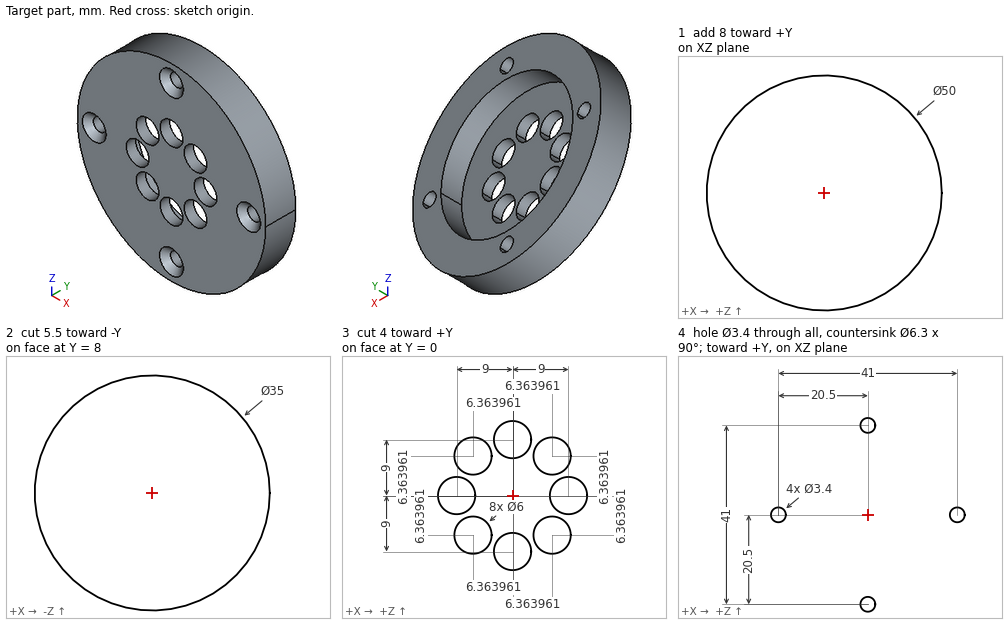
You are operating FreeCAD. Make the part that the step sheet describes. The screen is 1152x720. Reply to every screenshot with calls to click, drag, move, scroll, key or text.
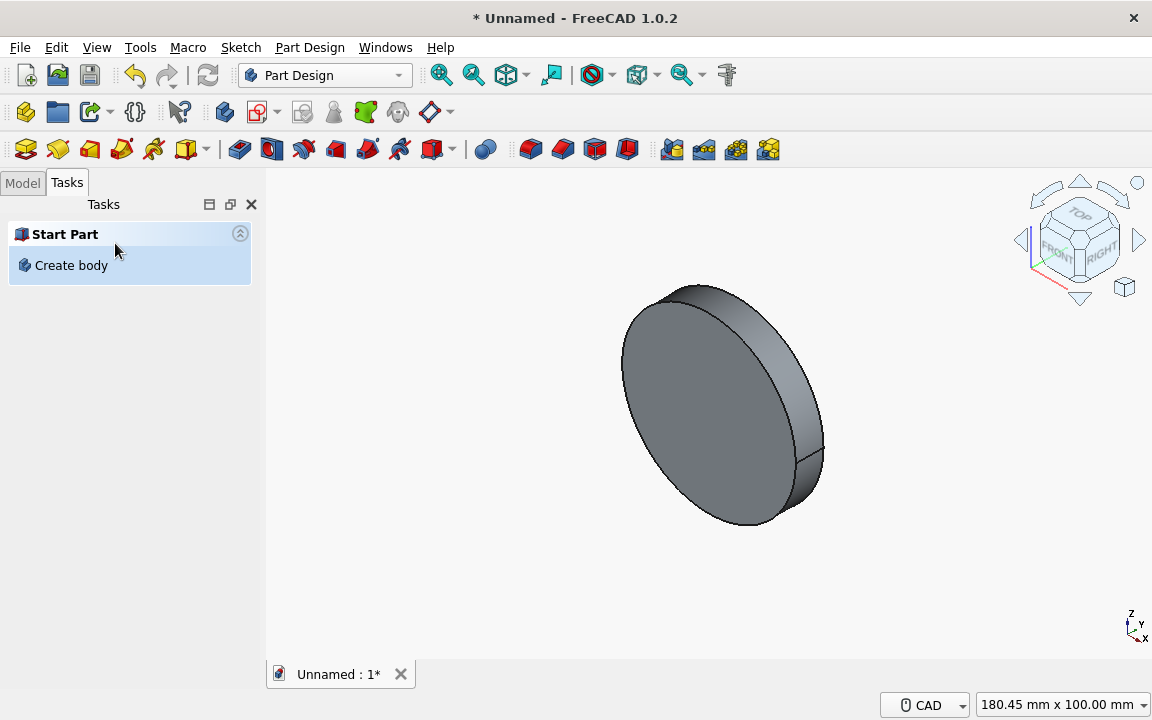
click(709, 412)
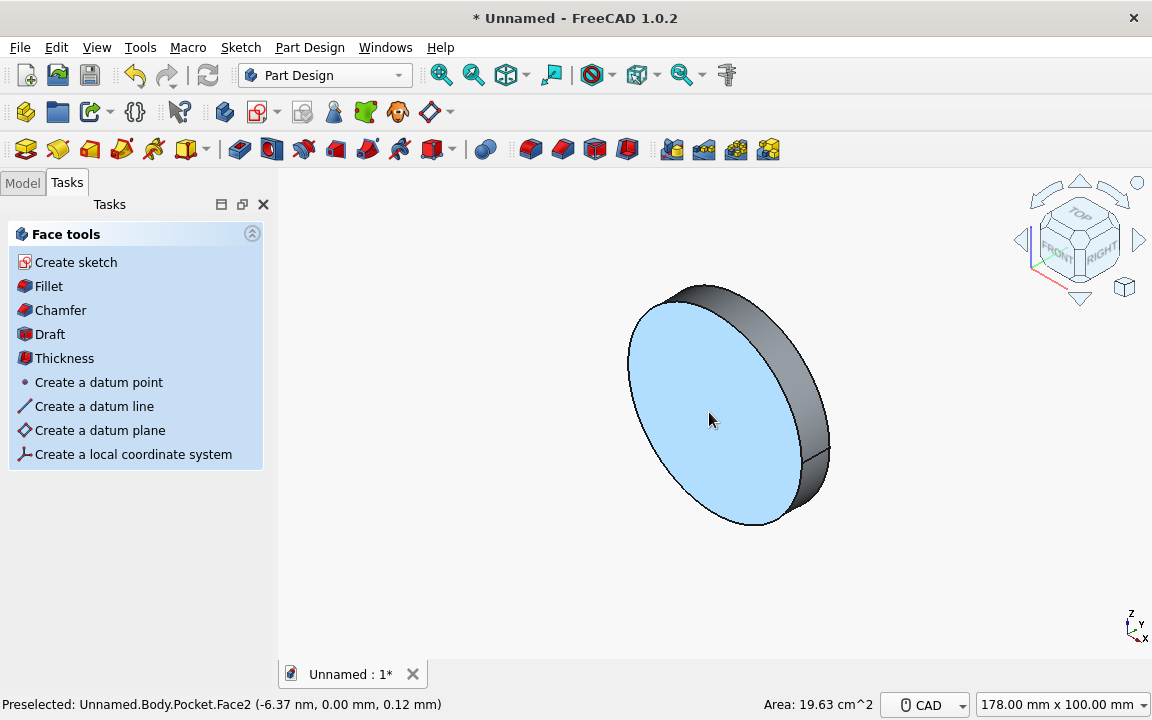
click(258, 112)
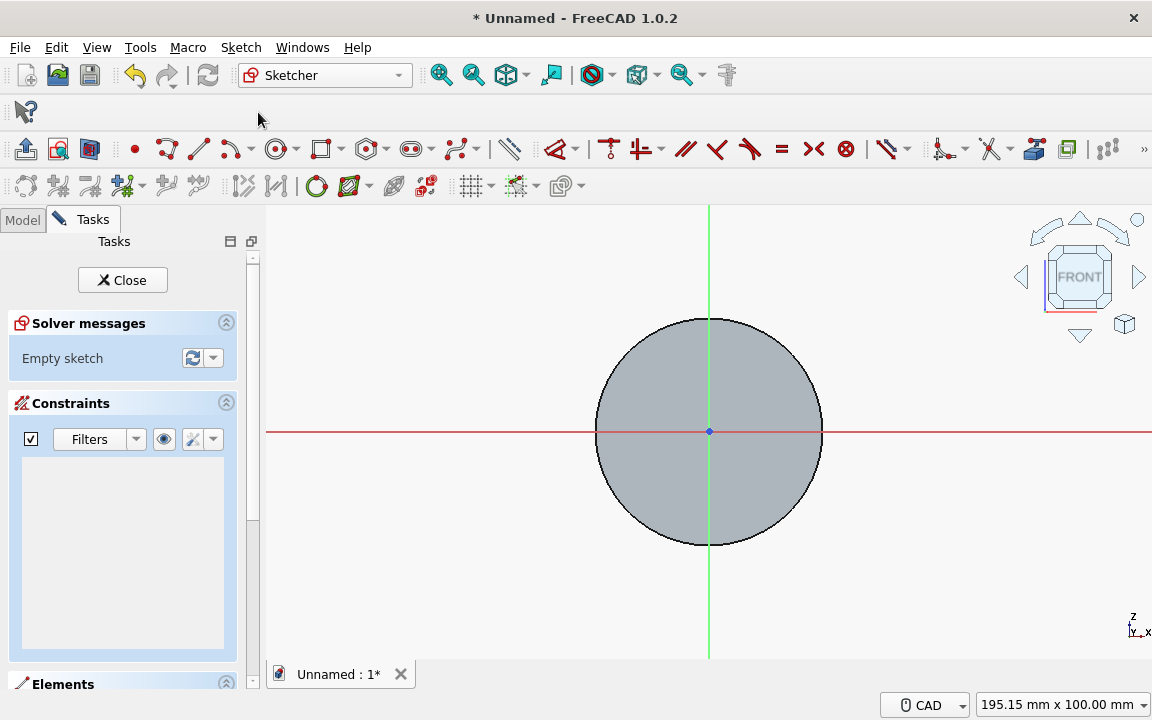
scroll(749, 432, up, 5)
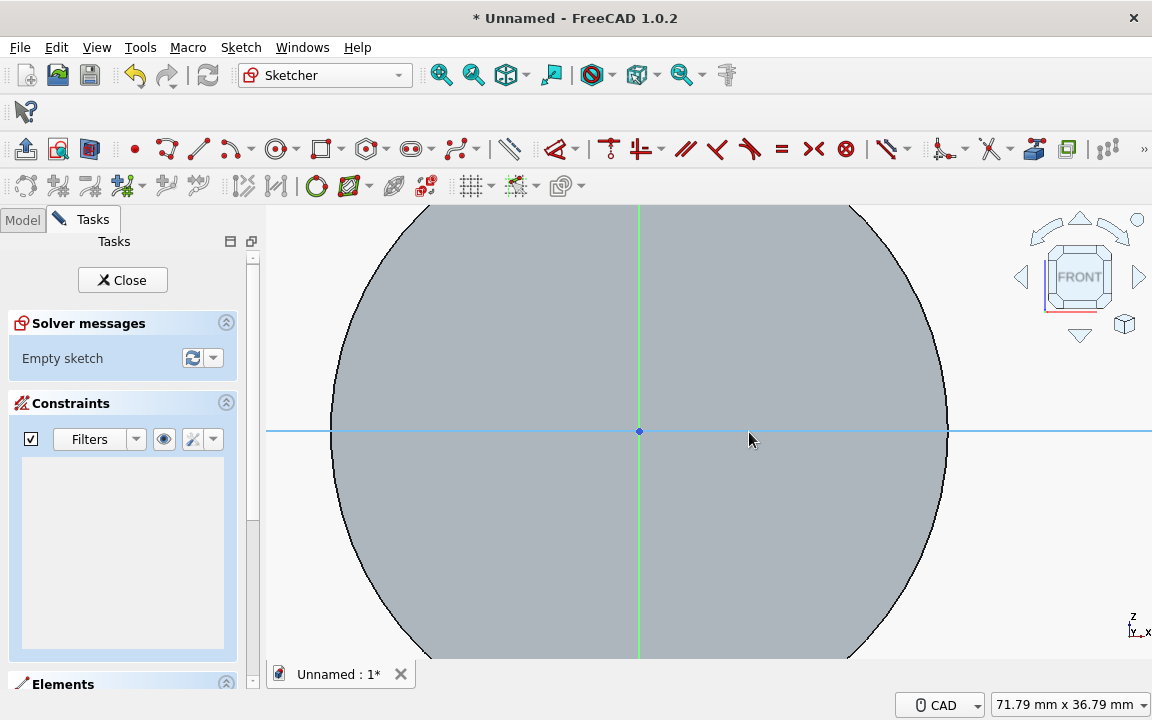
click(276, 150)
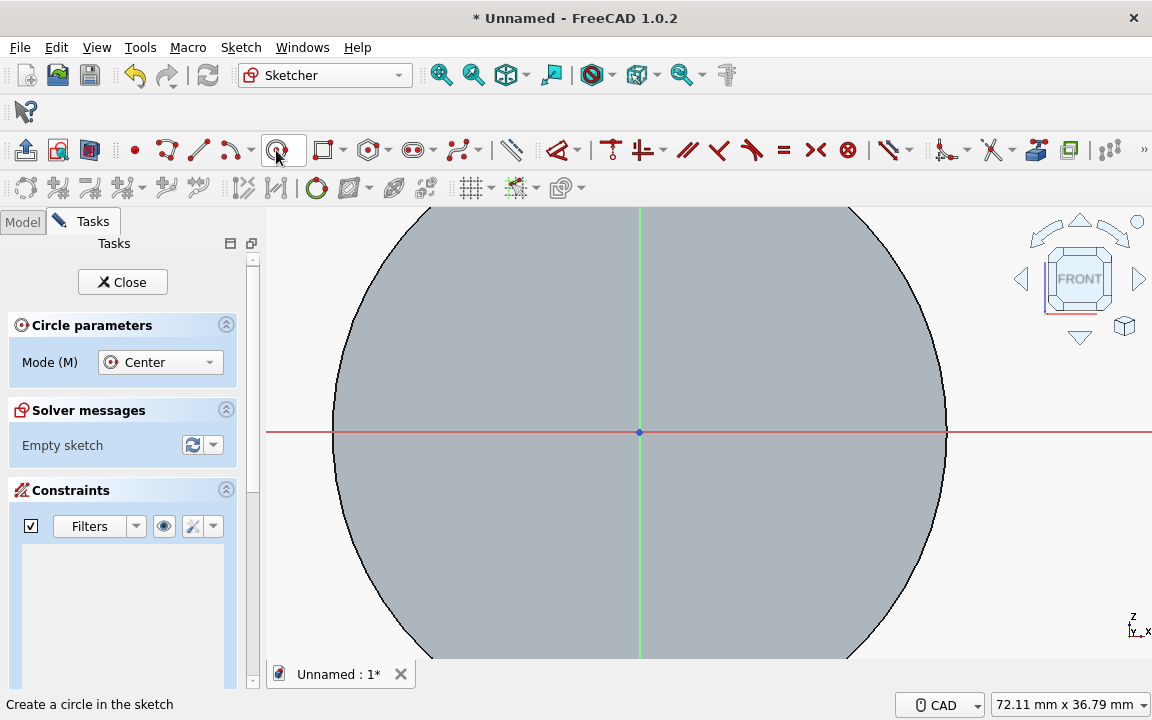
click(640, 543)
move(666, 517)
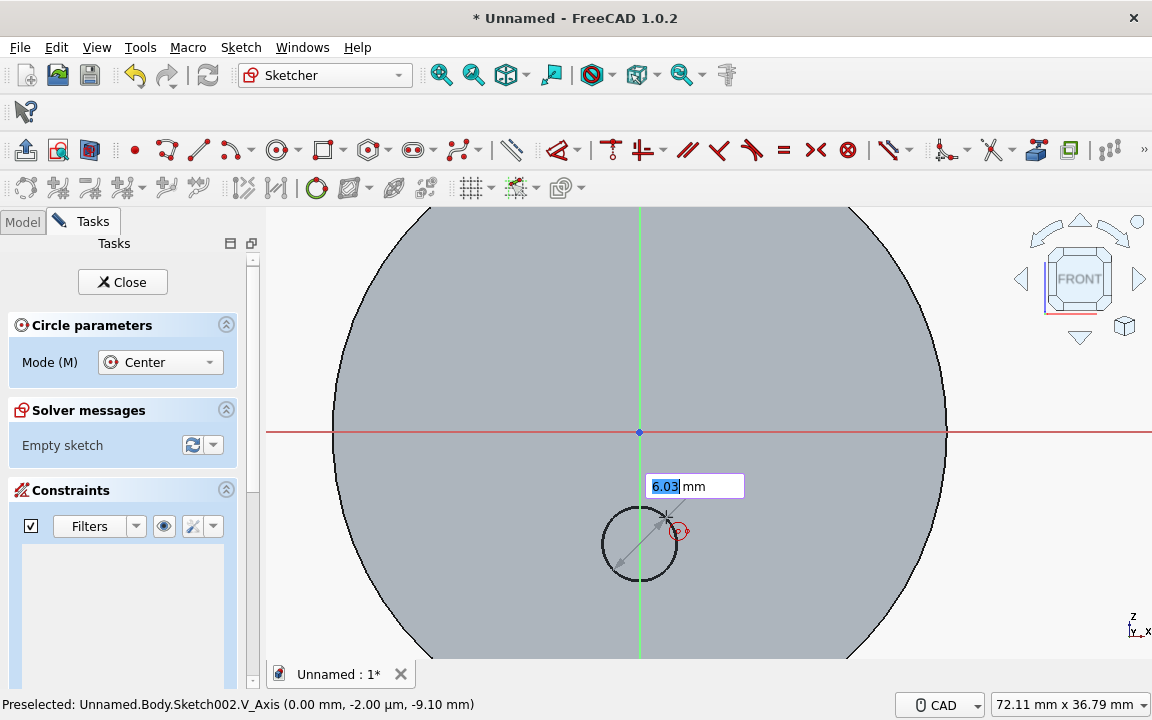
text(6)
key(Return)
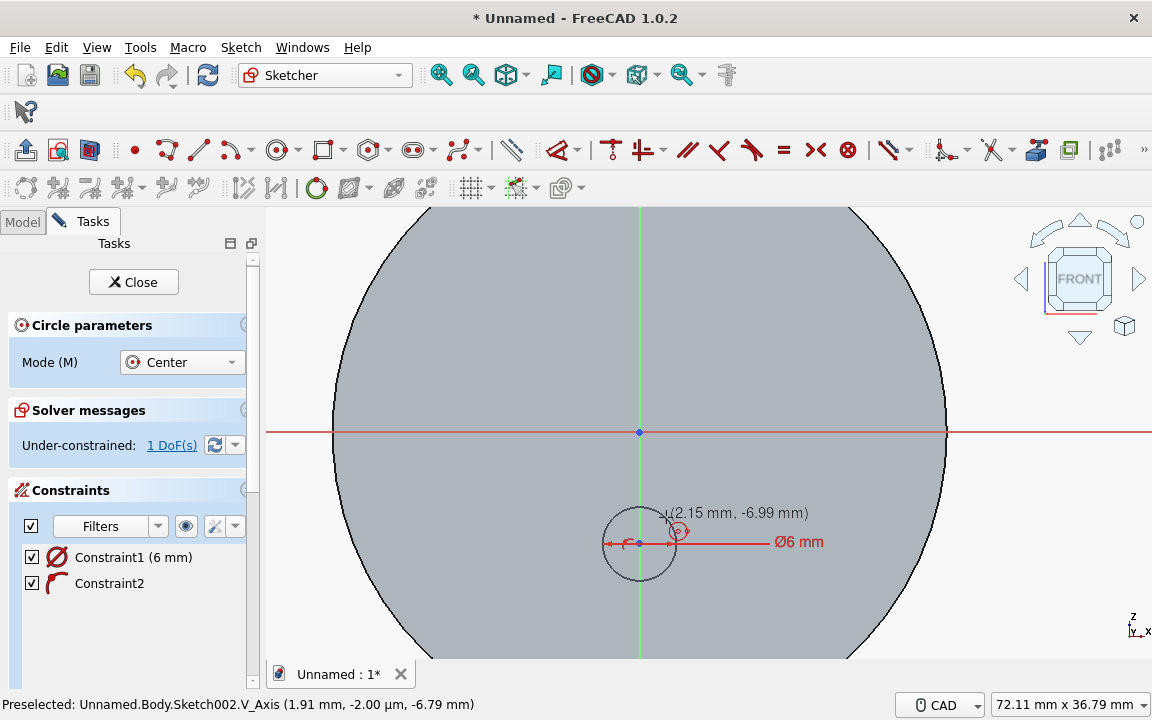
click(561, 510)
move(588, 484)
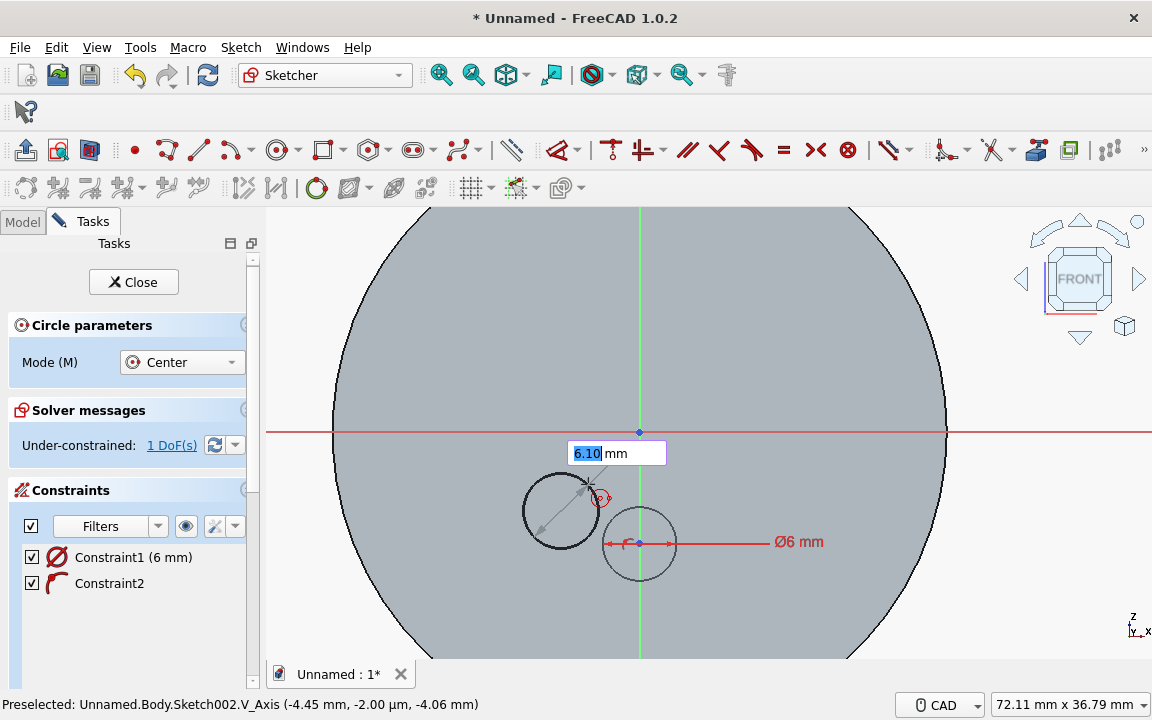
text(6)
key(Return)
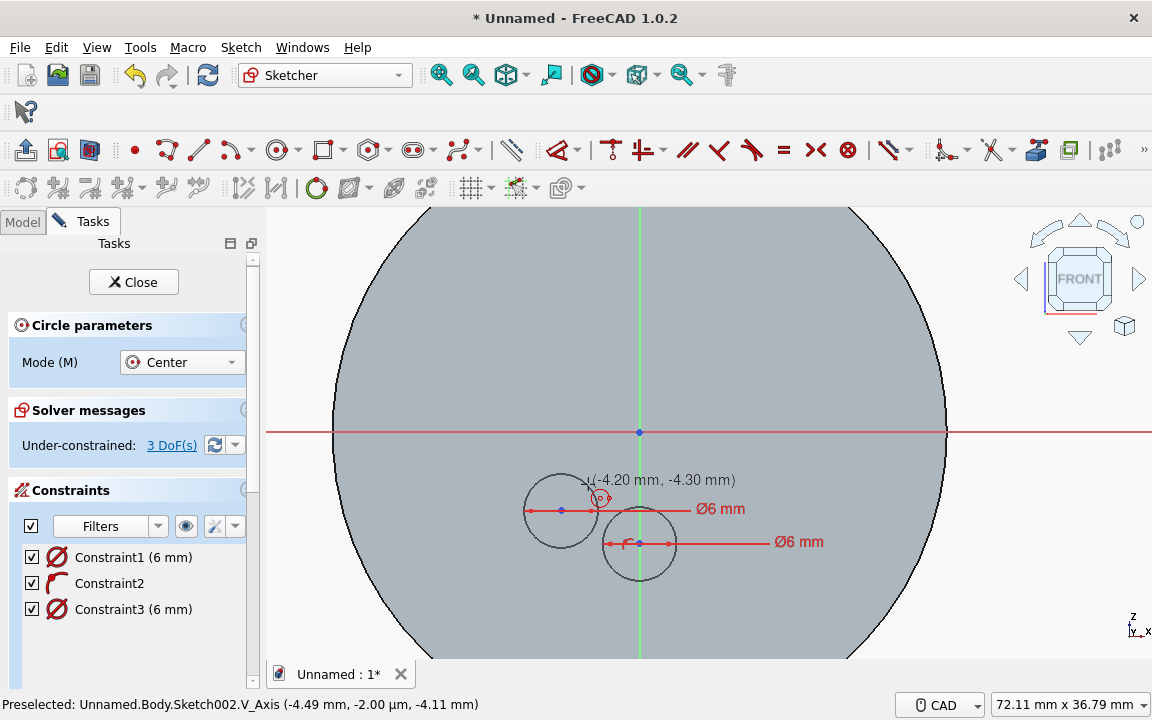
click(529, 432)
move(555, 406)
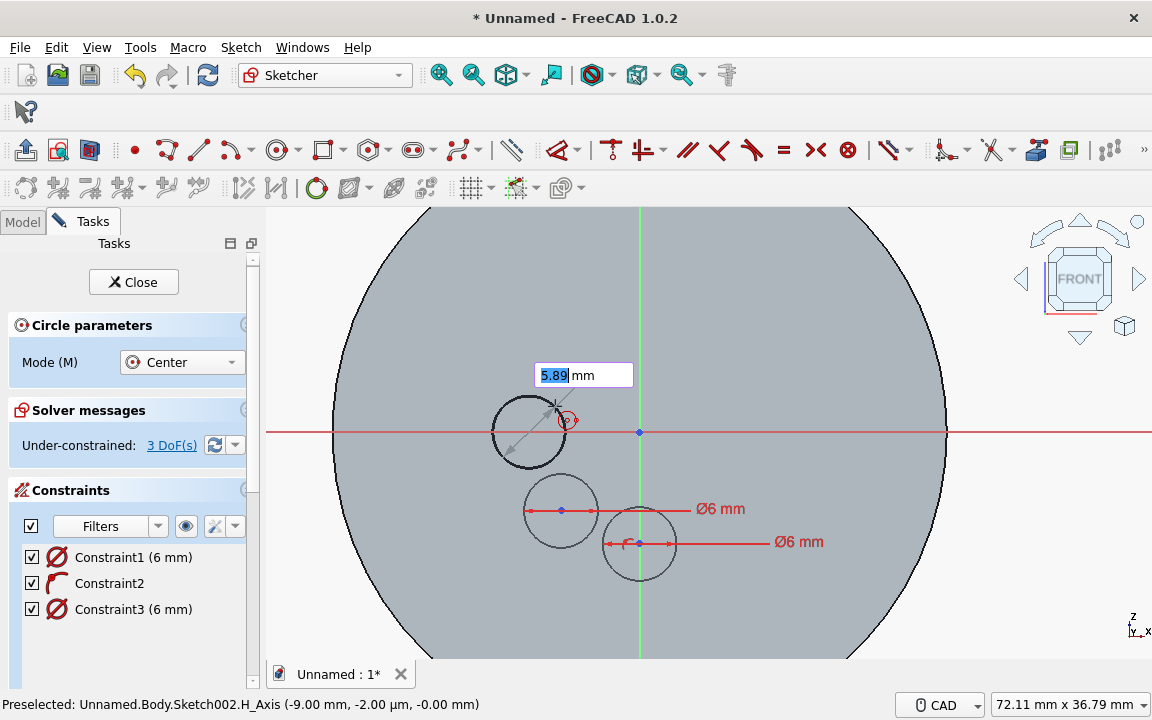
text(6)
key(Return)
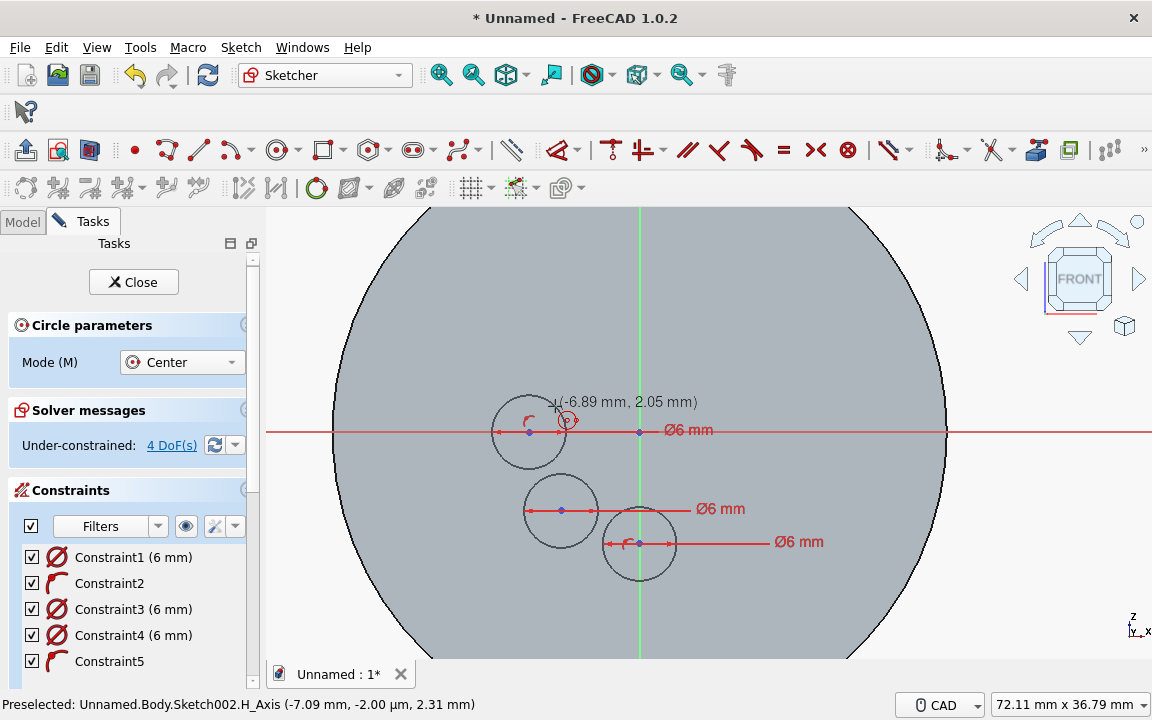
click(561, 354)
move(588, 328)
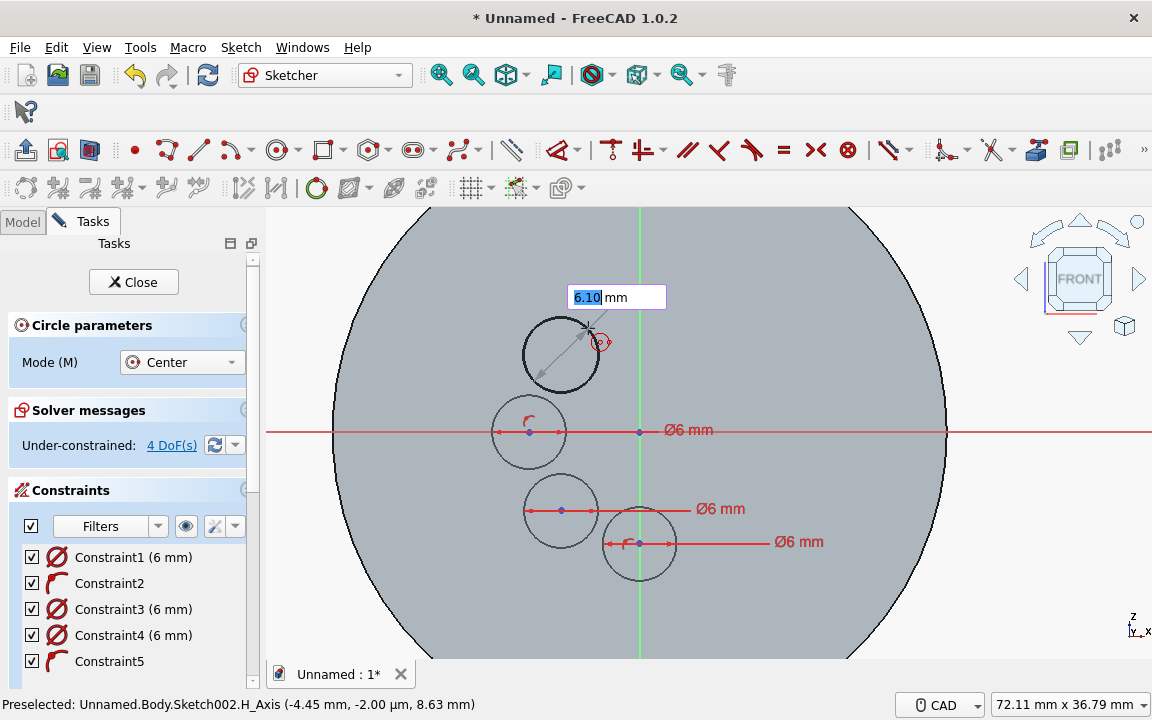
text(6)
key(Return)